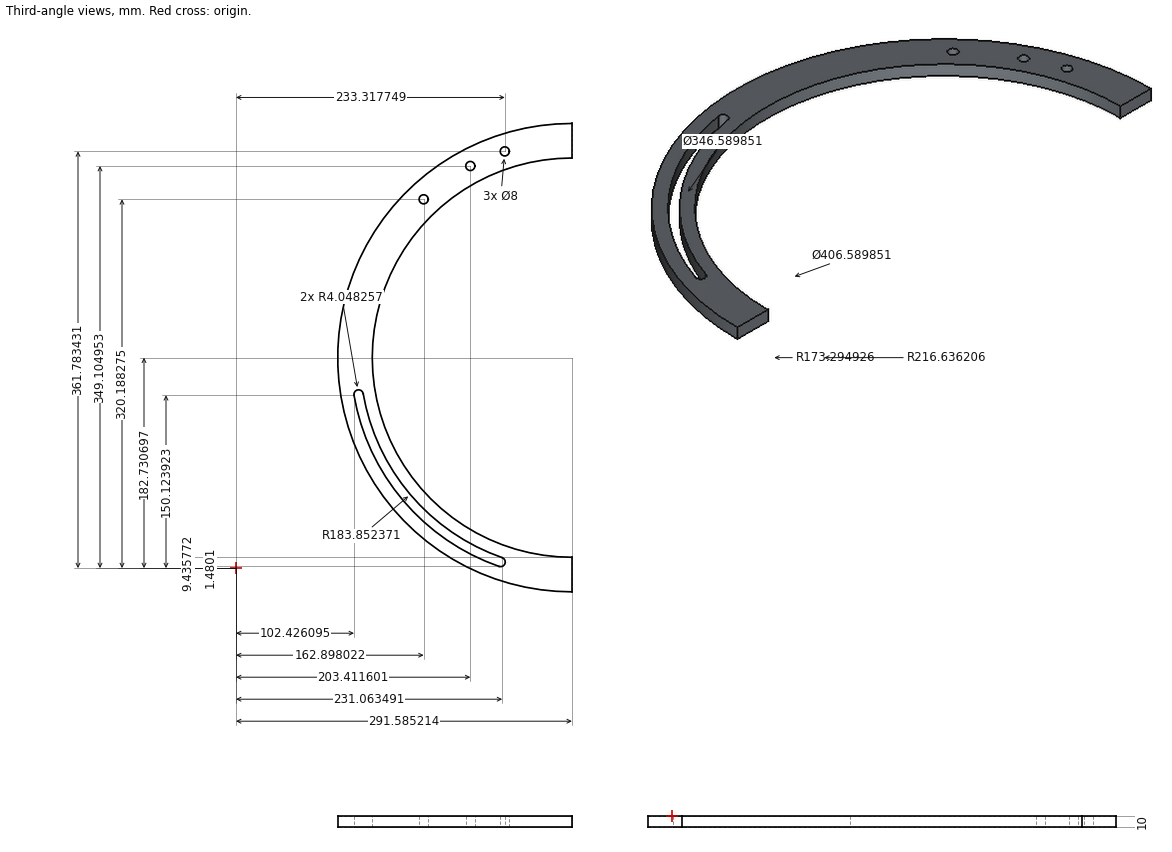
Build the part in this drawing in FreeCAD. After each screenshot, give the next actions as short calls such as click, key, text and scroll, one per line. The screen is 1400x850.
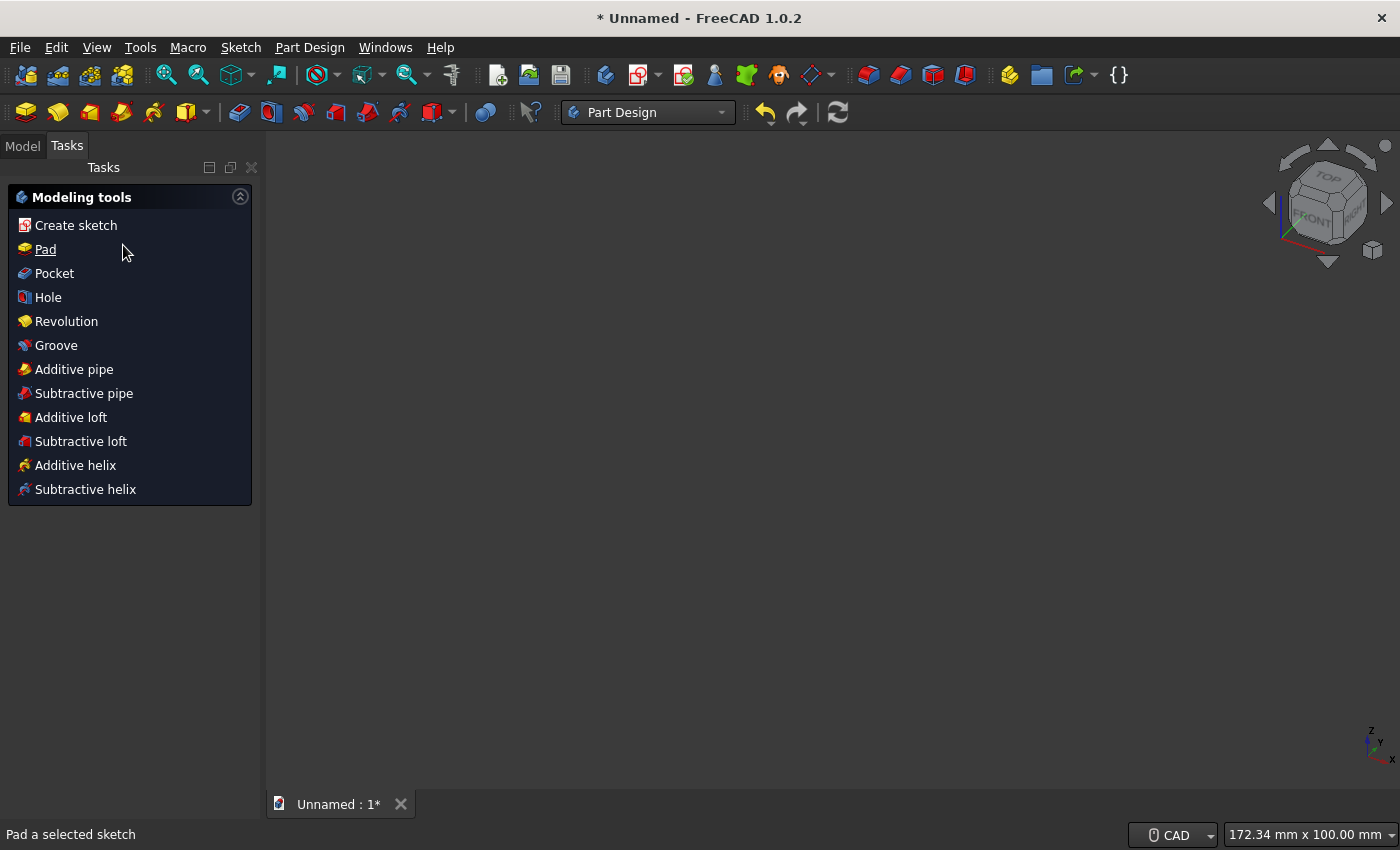
click(26, 112)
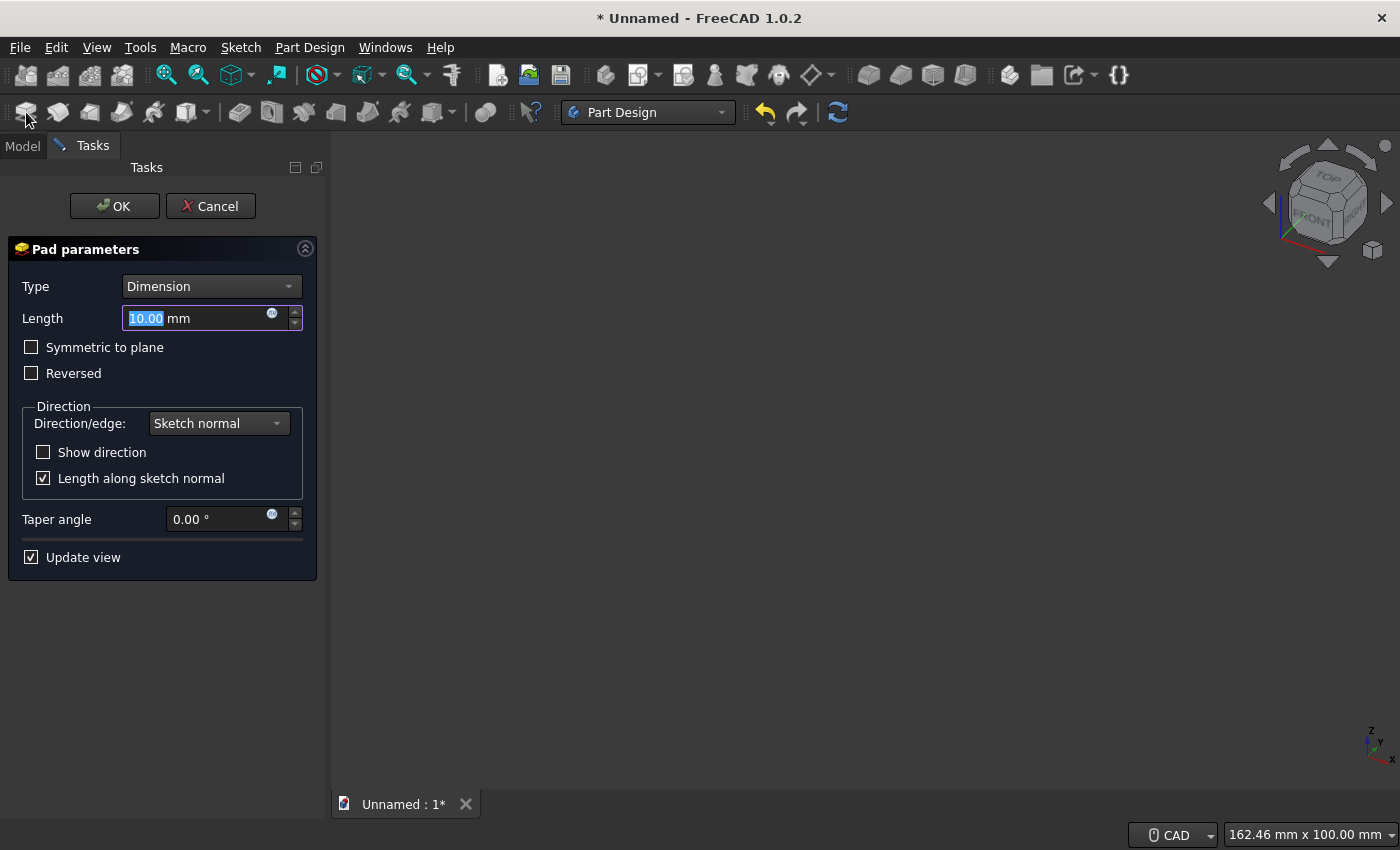
text(10)
key(Tab)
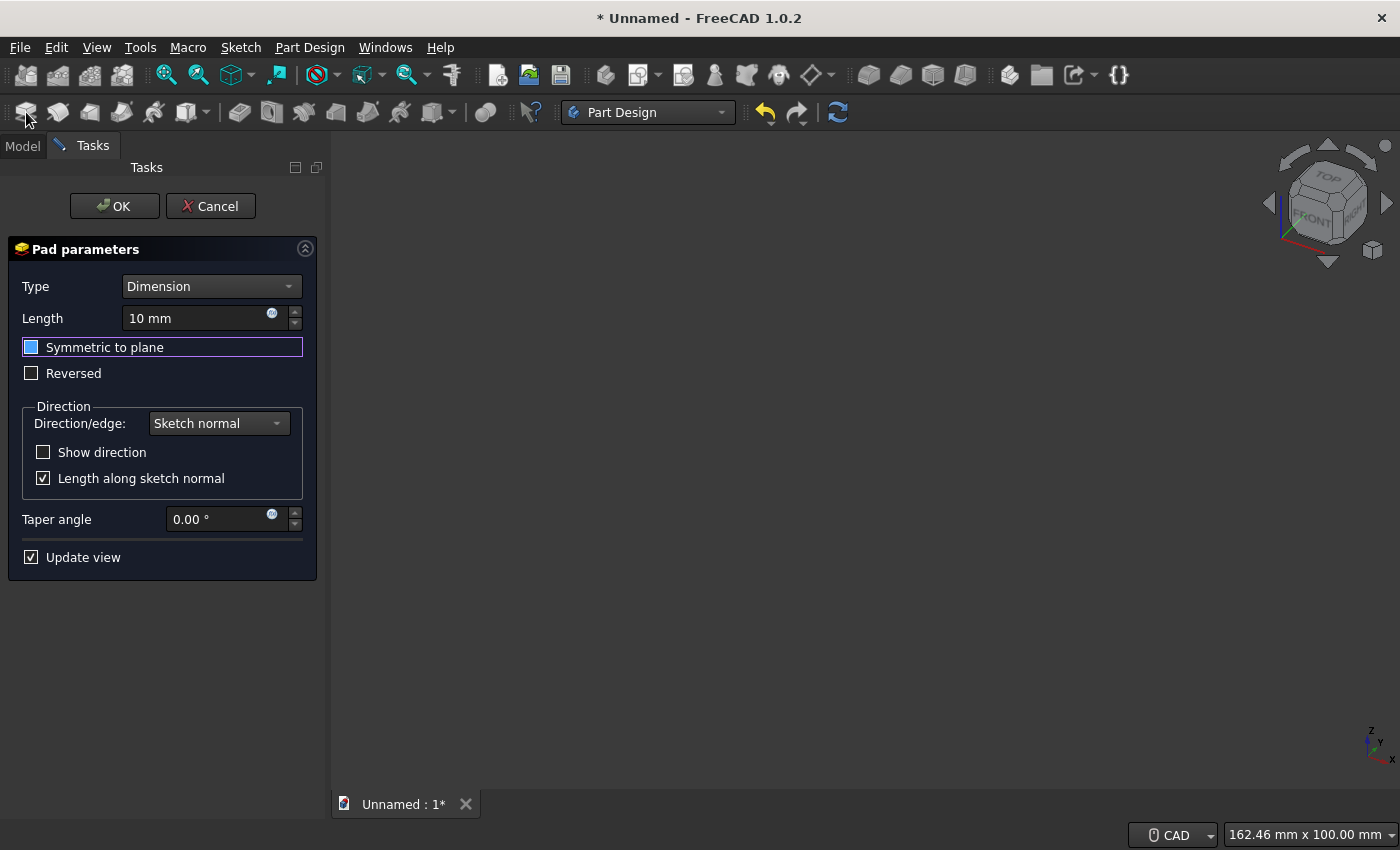
click(30, 373)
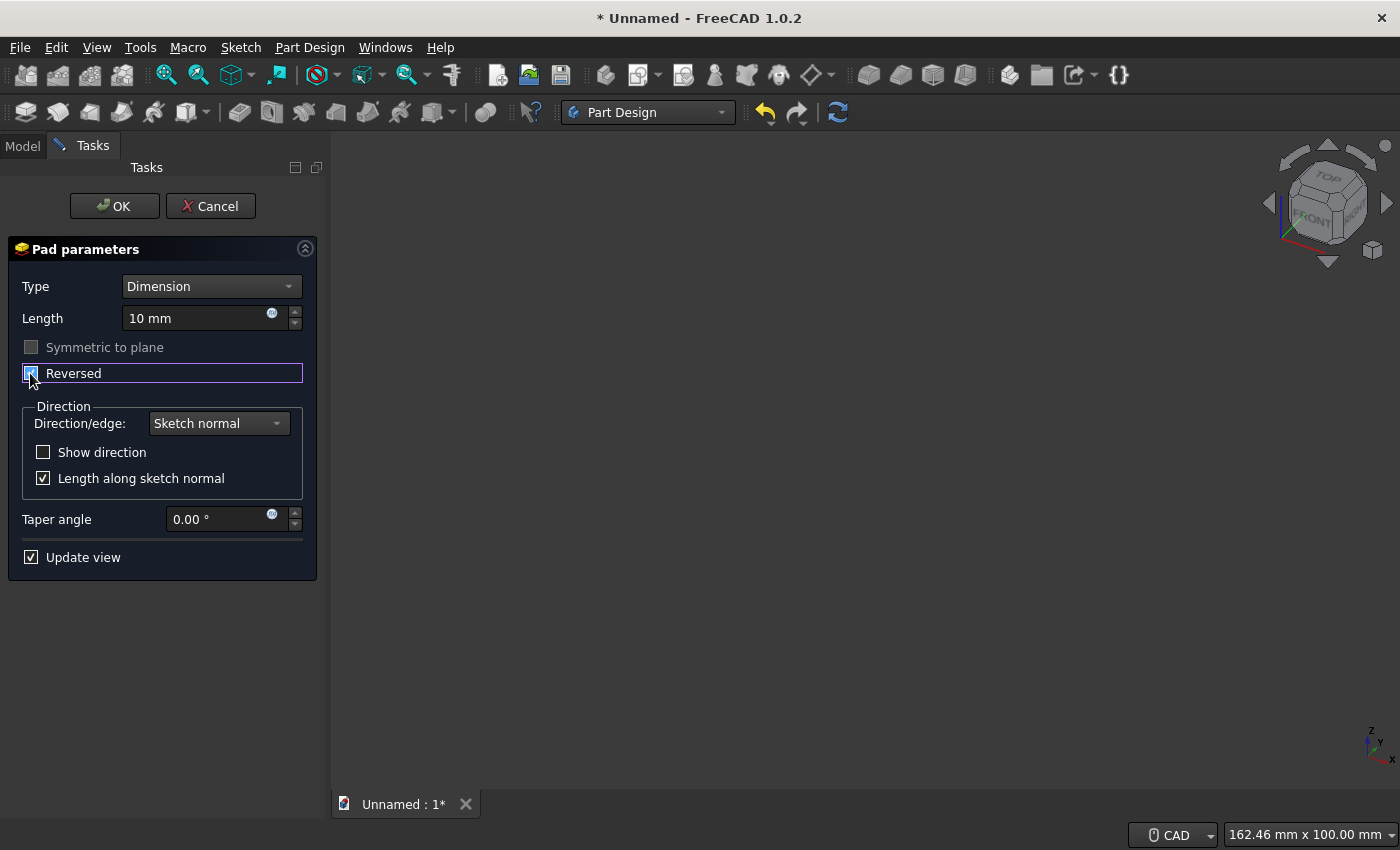
click(115, 206)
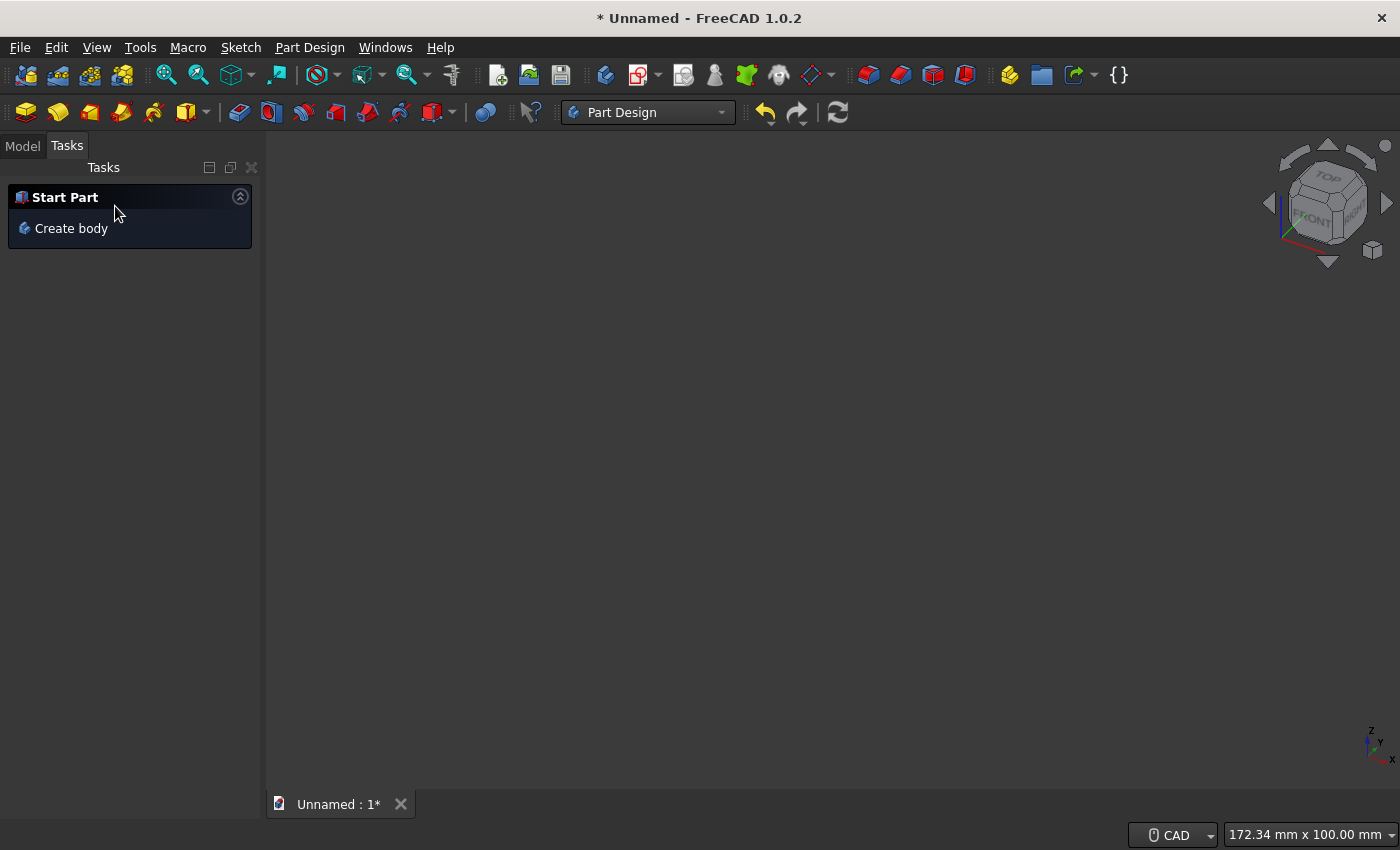
click(168, 76)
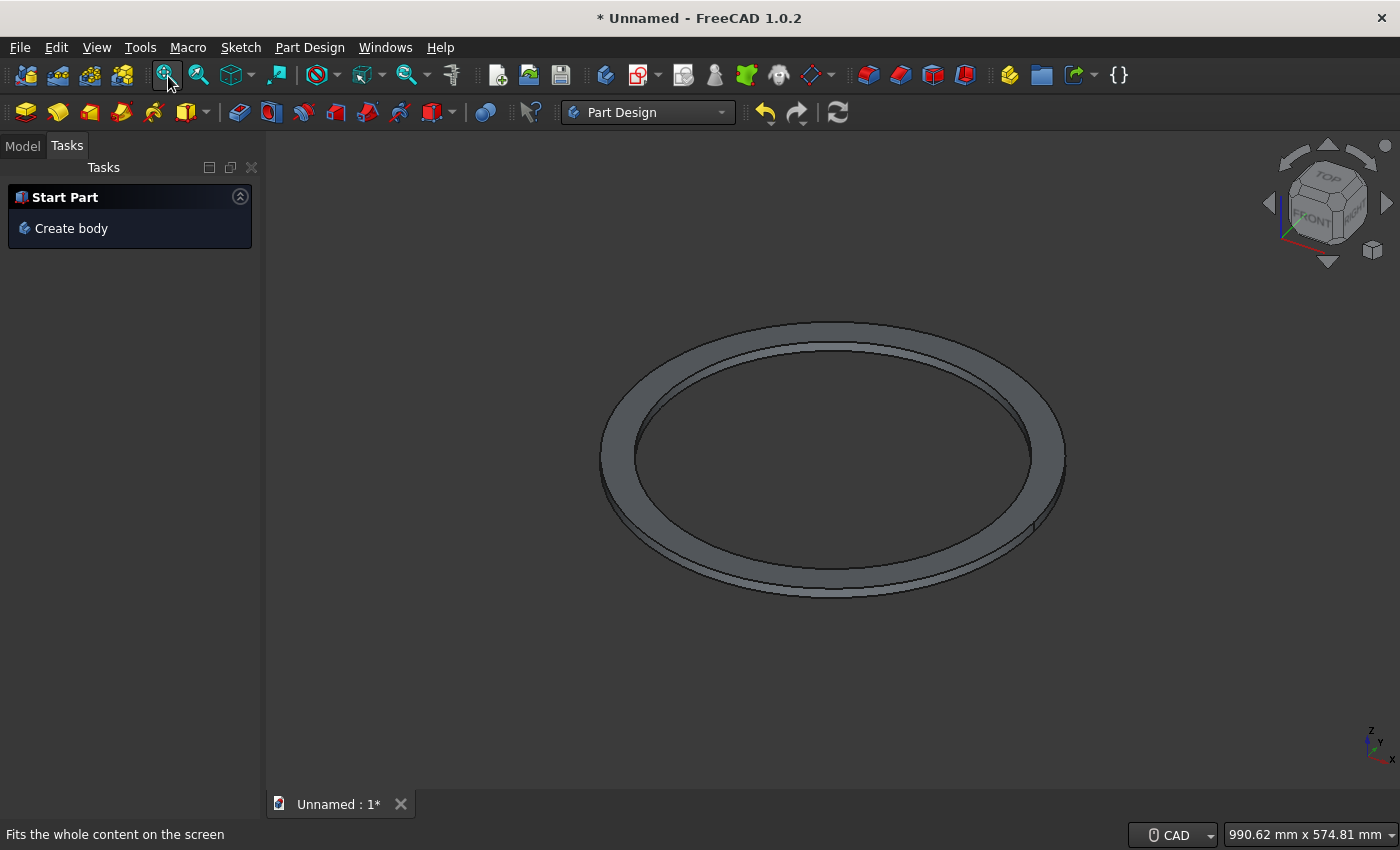
click(23, 145)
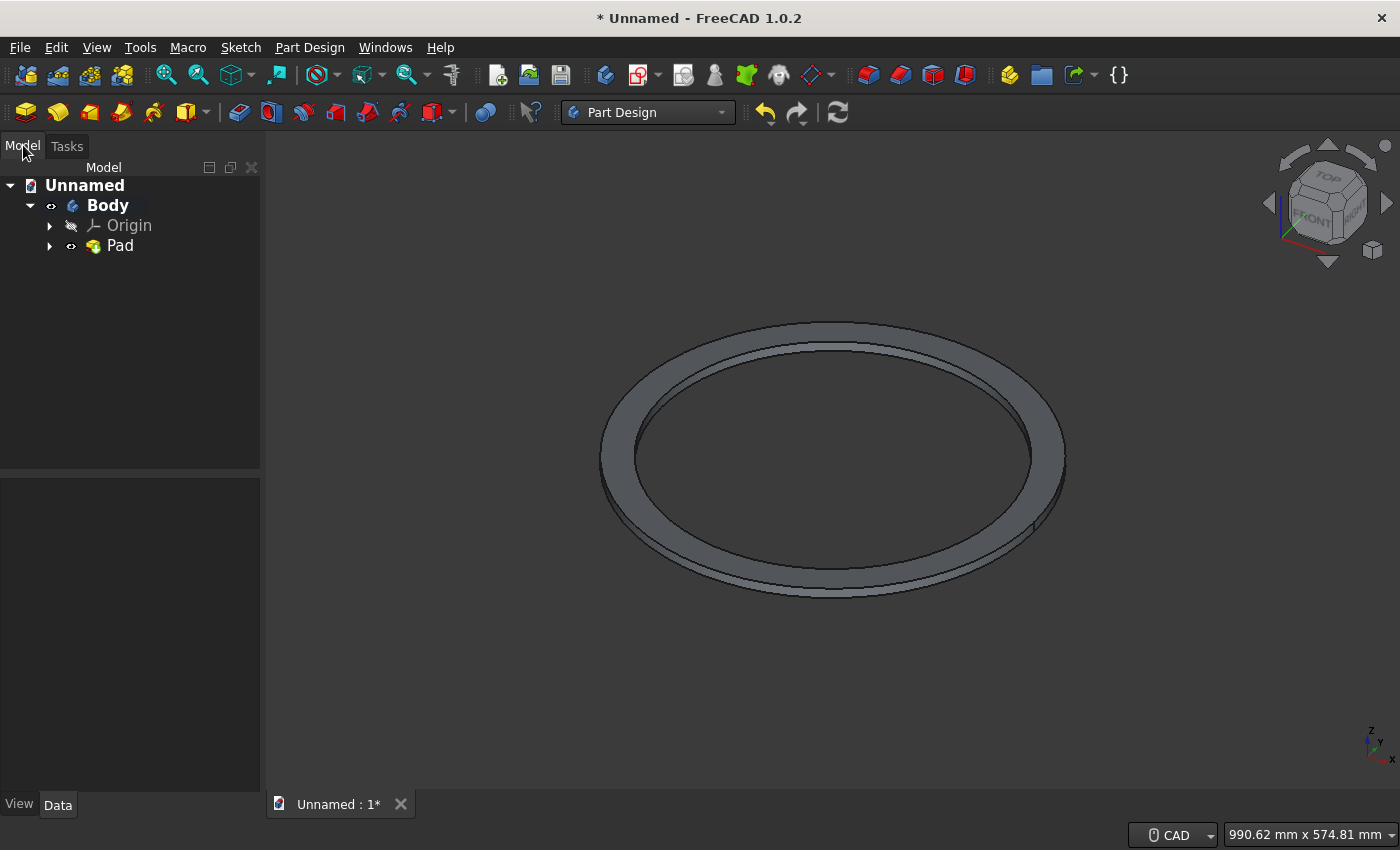
click(50, 226)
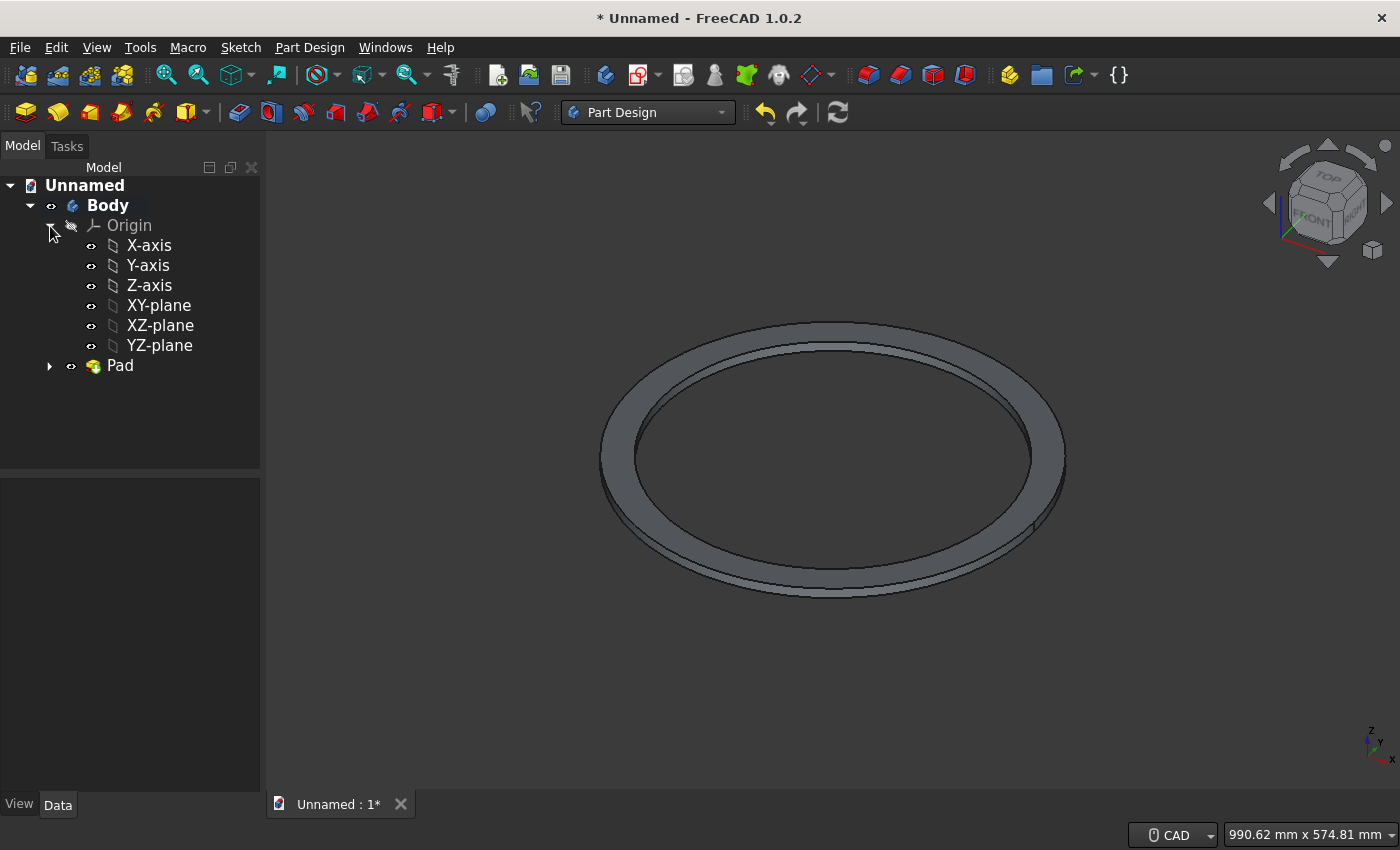
click(136, 306)